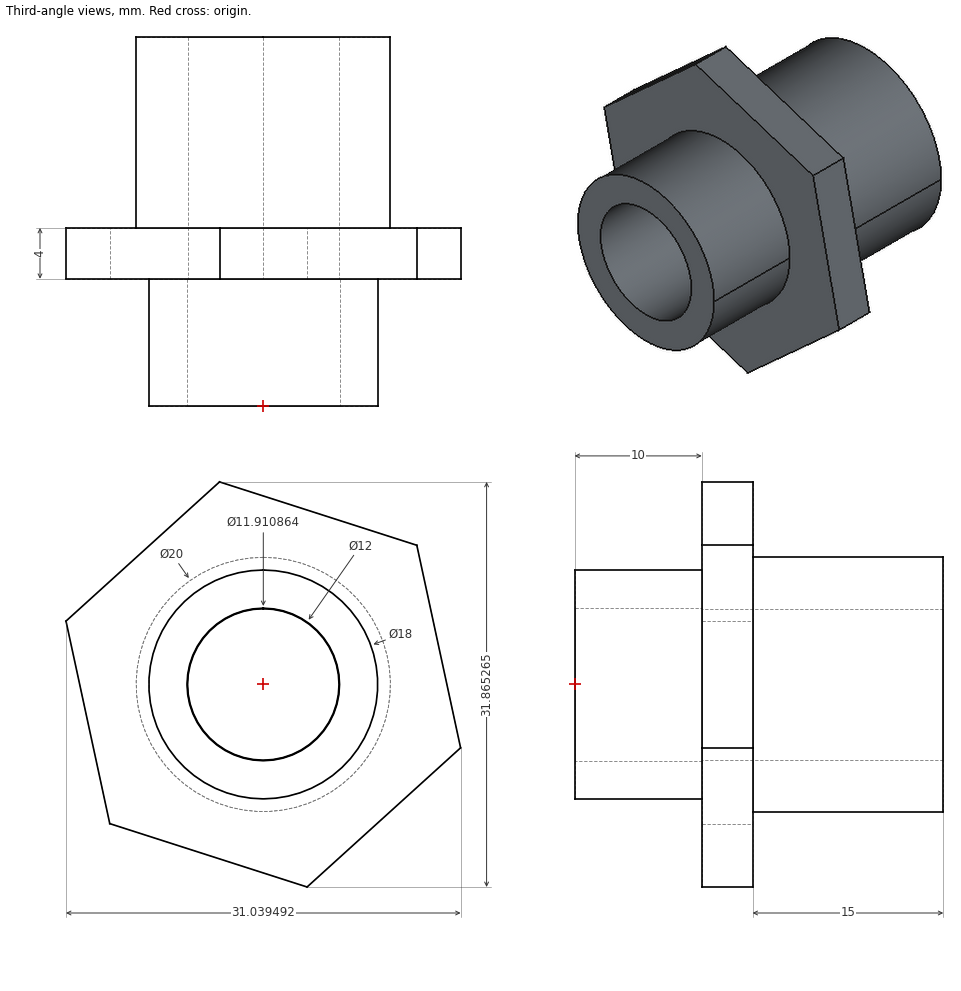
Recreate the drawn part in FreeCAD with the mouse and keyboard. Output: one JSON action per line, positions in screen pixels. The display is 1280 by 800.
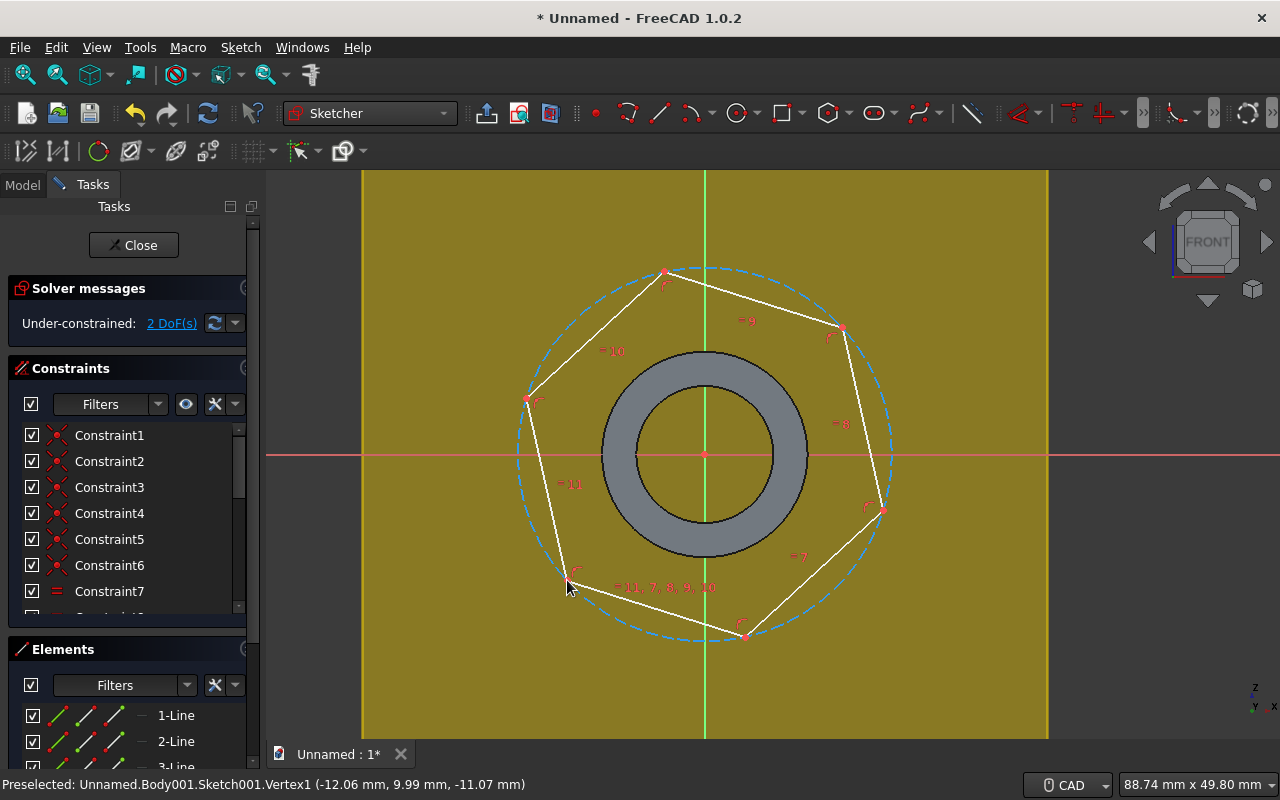
{"action": "left_click", "coordinate": [738, 114]}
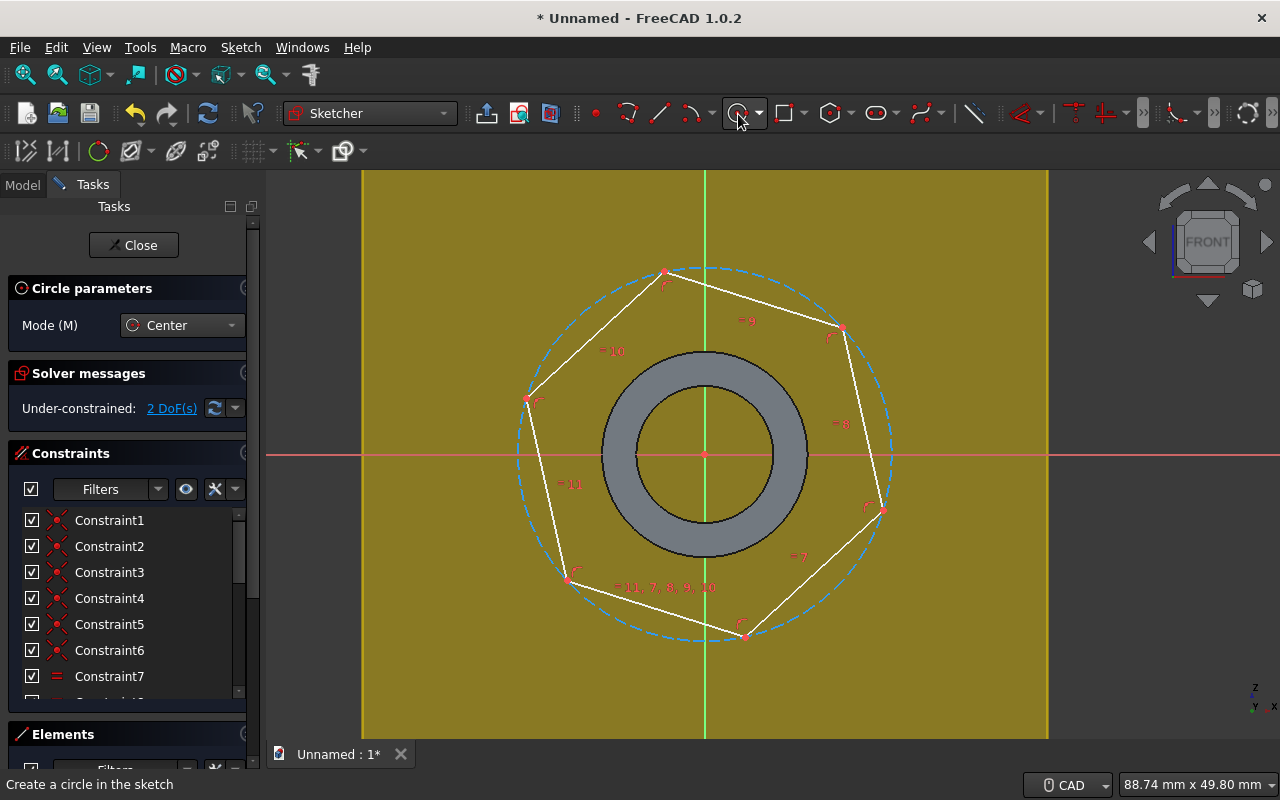
{"action": "left_click", "coordinate": [705, 455]}
{"action": "mouse_move", "coordinate": [753, 406]}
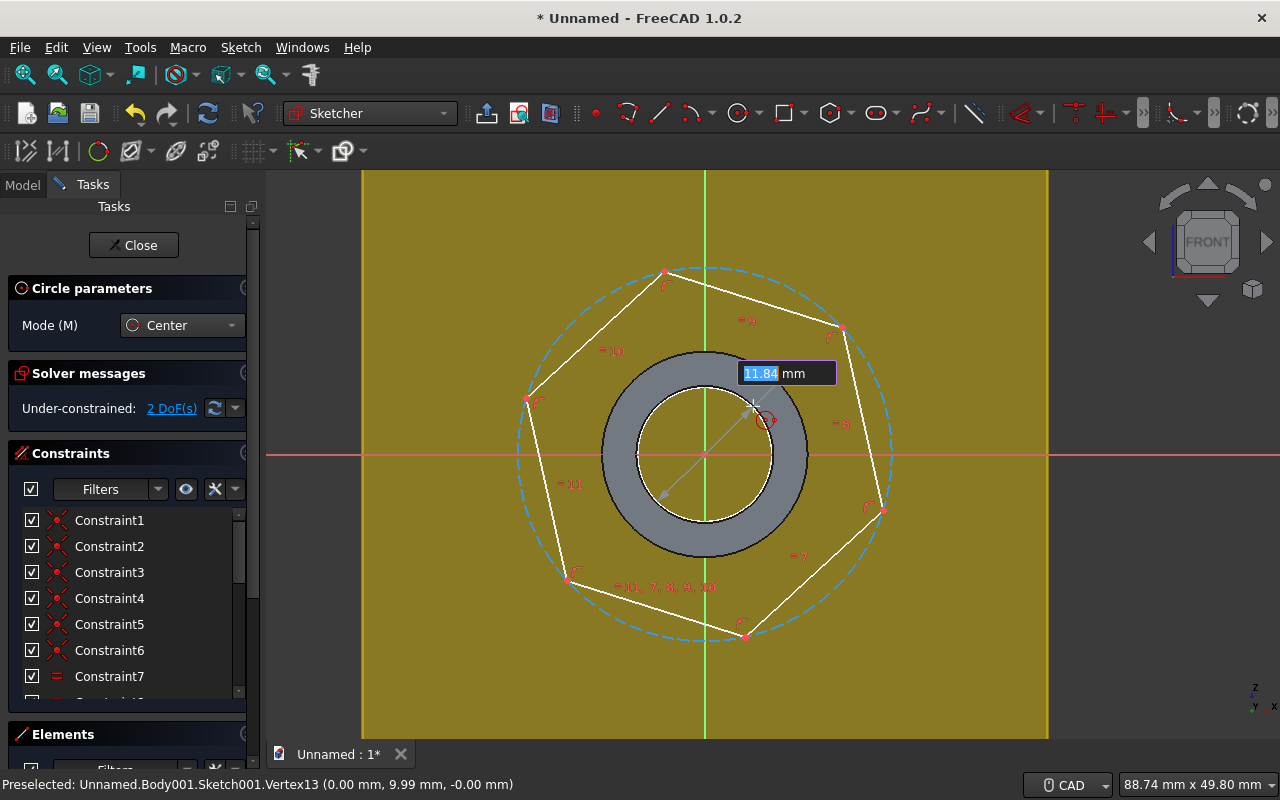
{"action": "type", "text": "11.910864"}
{"action": "key", "text": "Return"}
{"action": "key", "text": "Escape"}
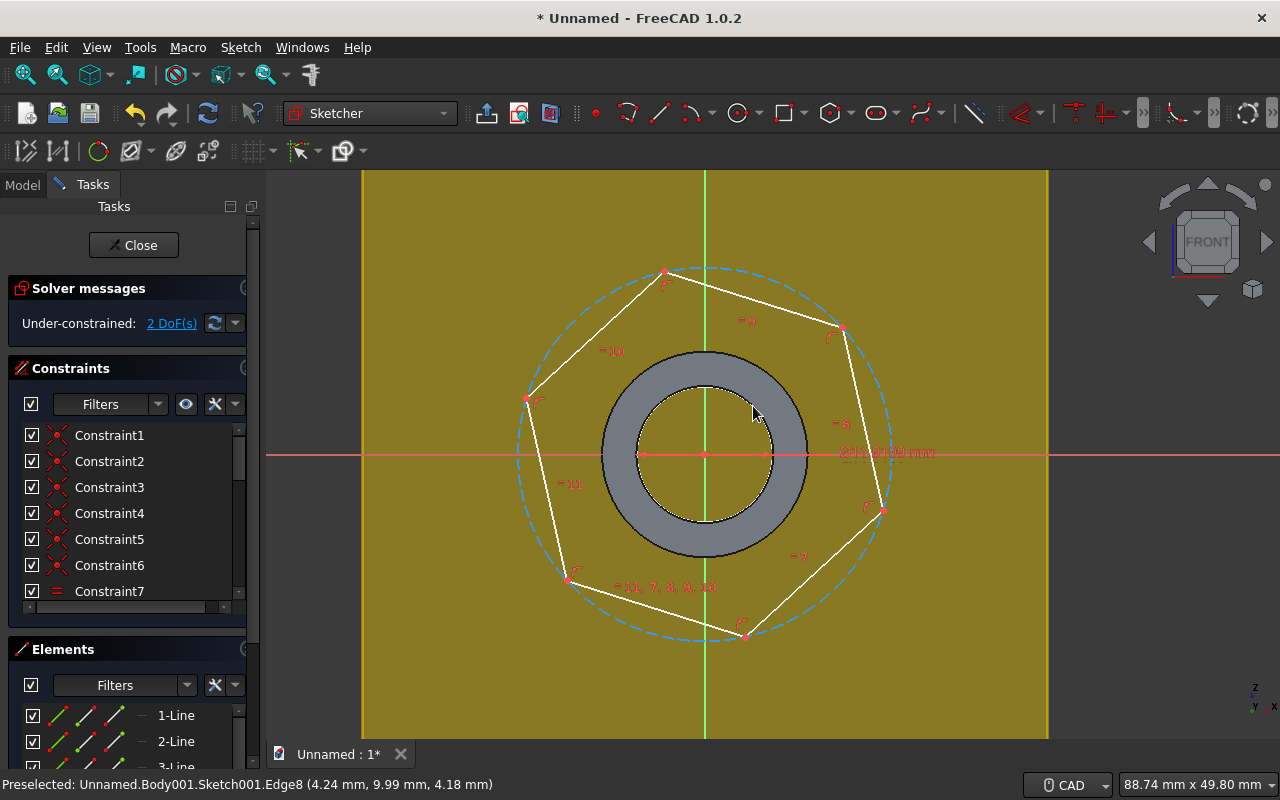
{"action": "left_click", "coordinate": [1020, 114]}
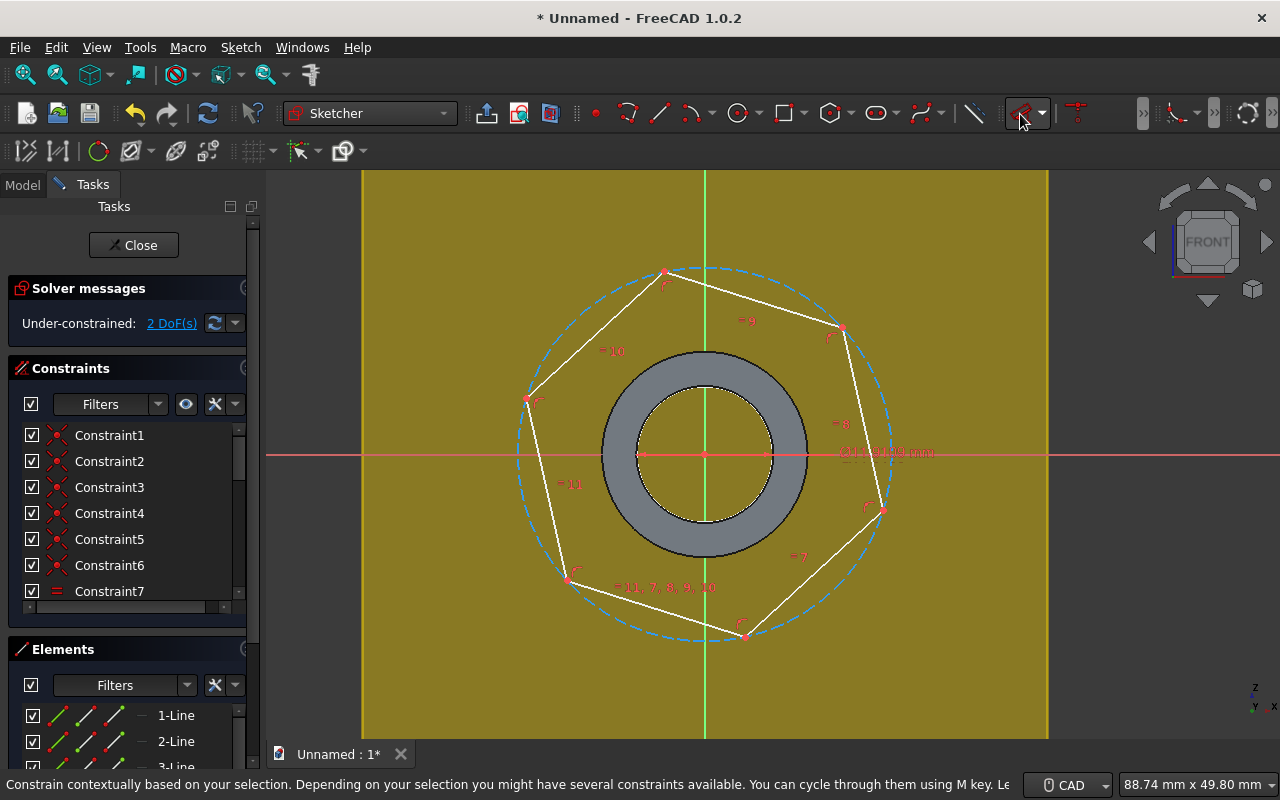
{"action": "left_click", "coordinate": [526, 398]}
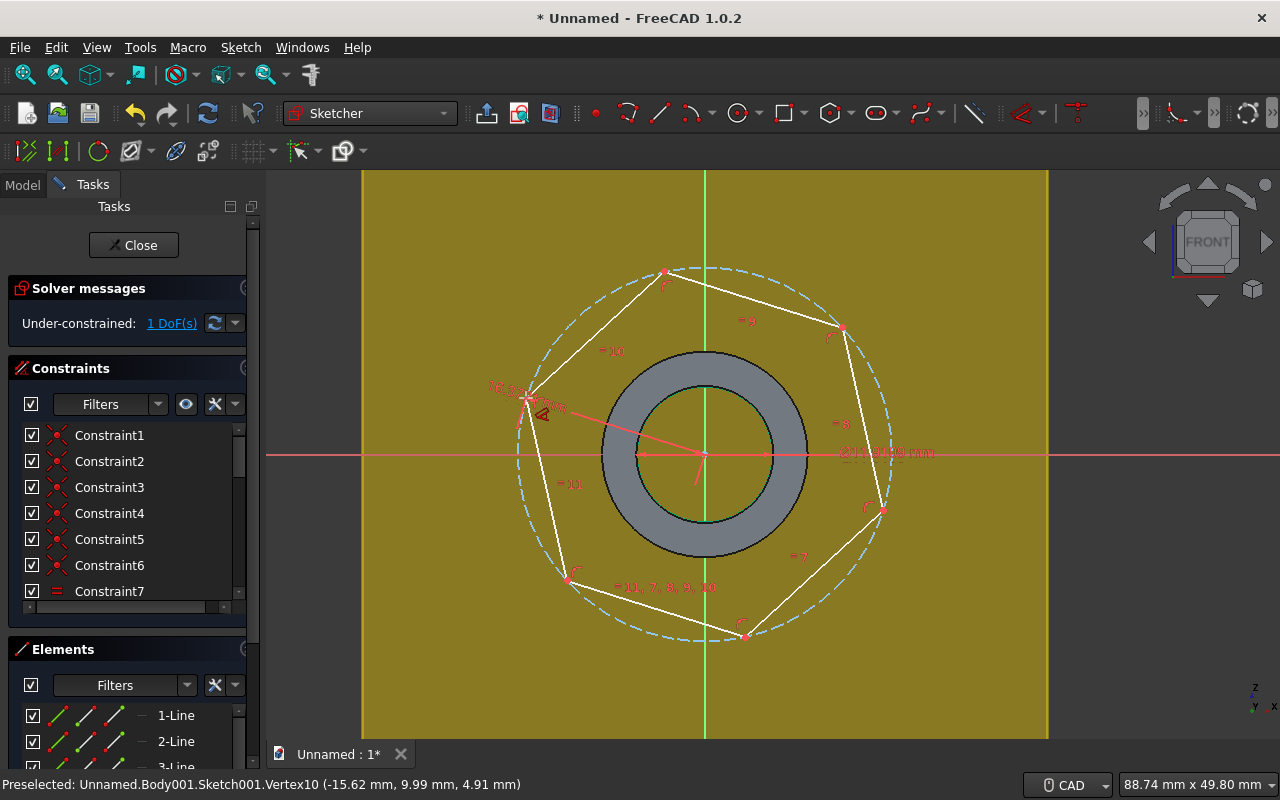
{"action": "left_click", "coordinate": [883, 511]}
{"action": "left_click", "coordinate": [623, 364]}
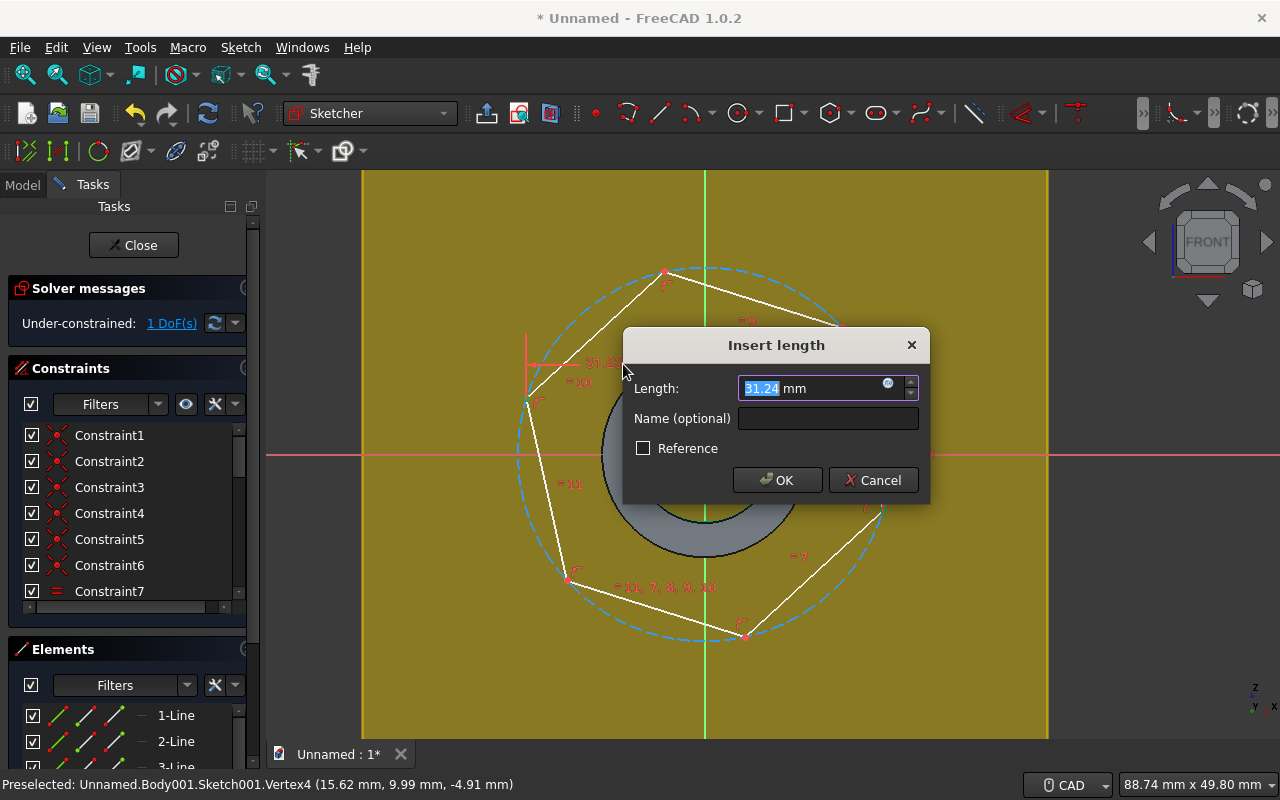
{"action": "type", "text": "31.039492"}
{"action": "key", "text": "Return"}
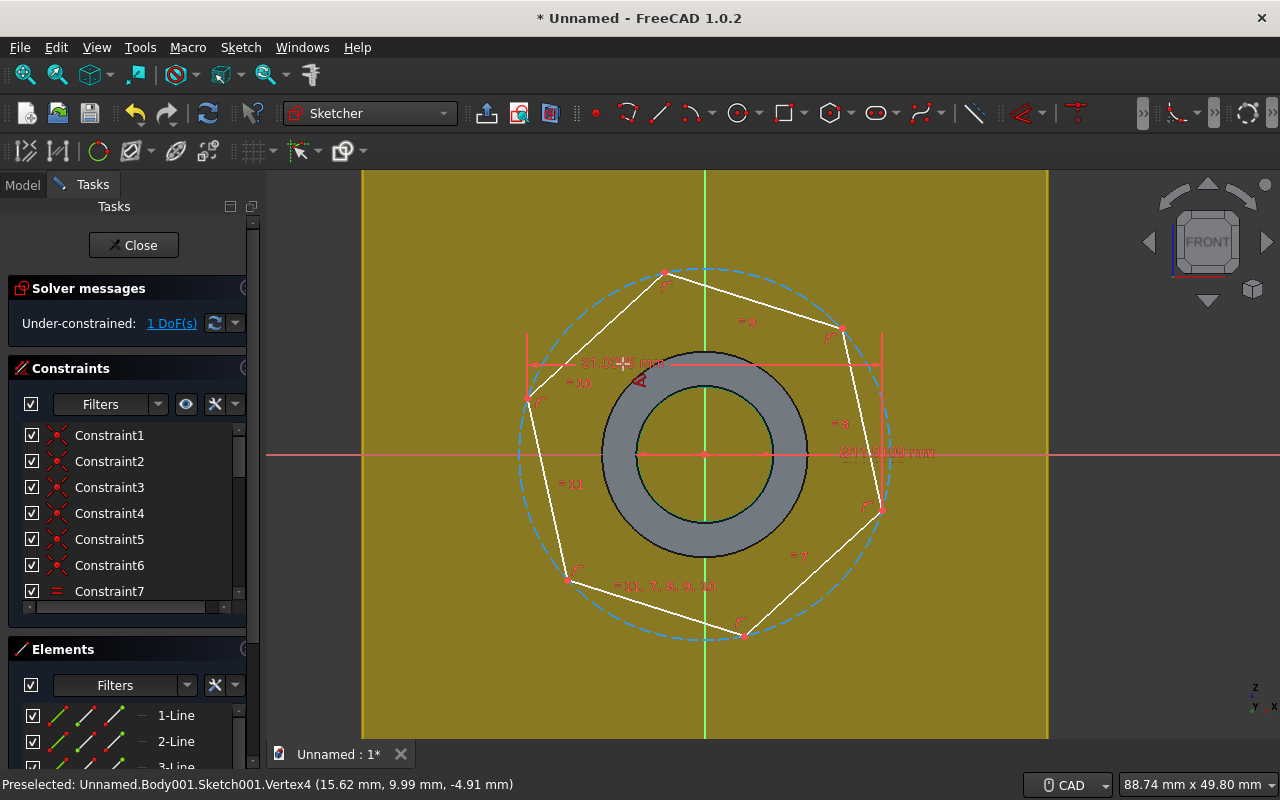
{"action": "left_click", "coordinate": [745, 636]}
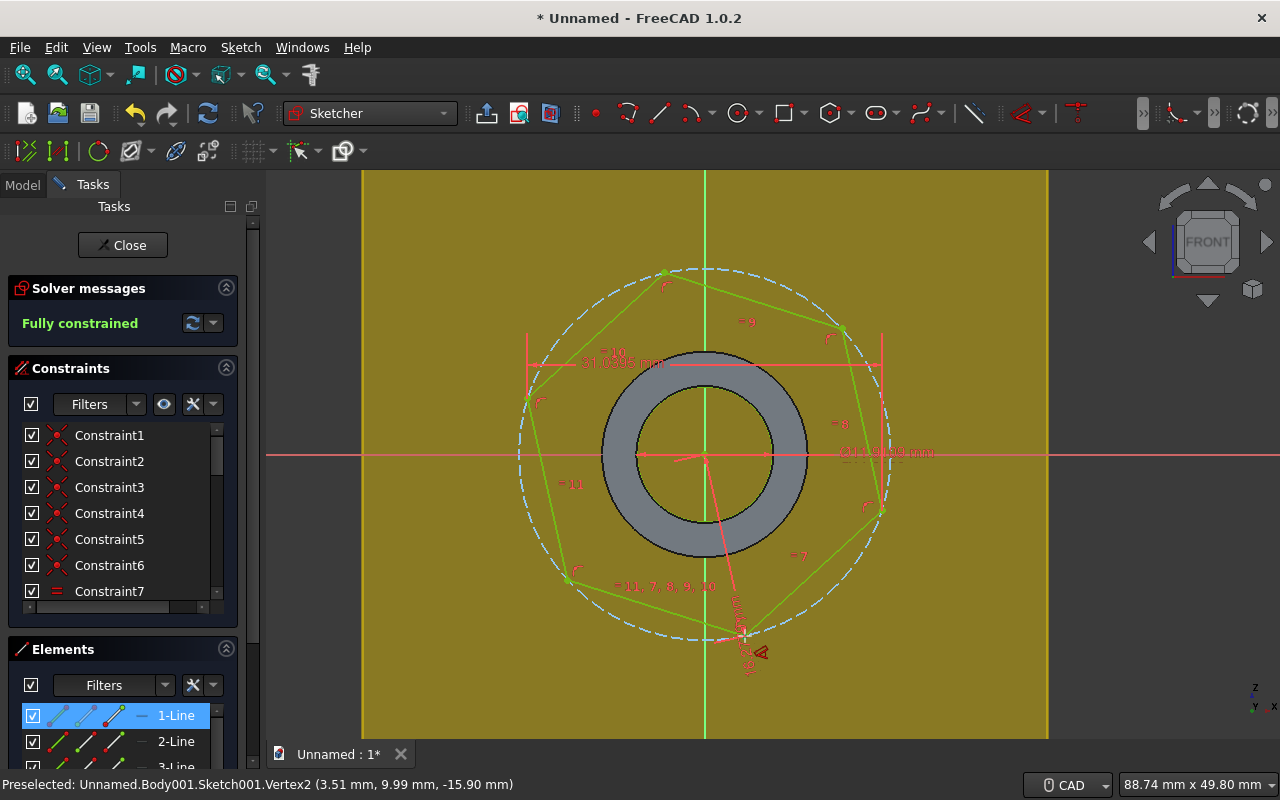
{"action": "left_click", "coordinate": [665, 273]}
{"action": "left_click", "coordinate": [779, 371]}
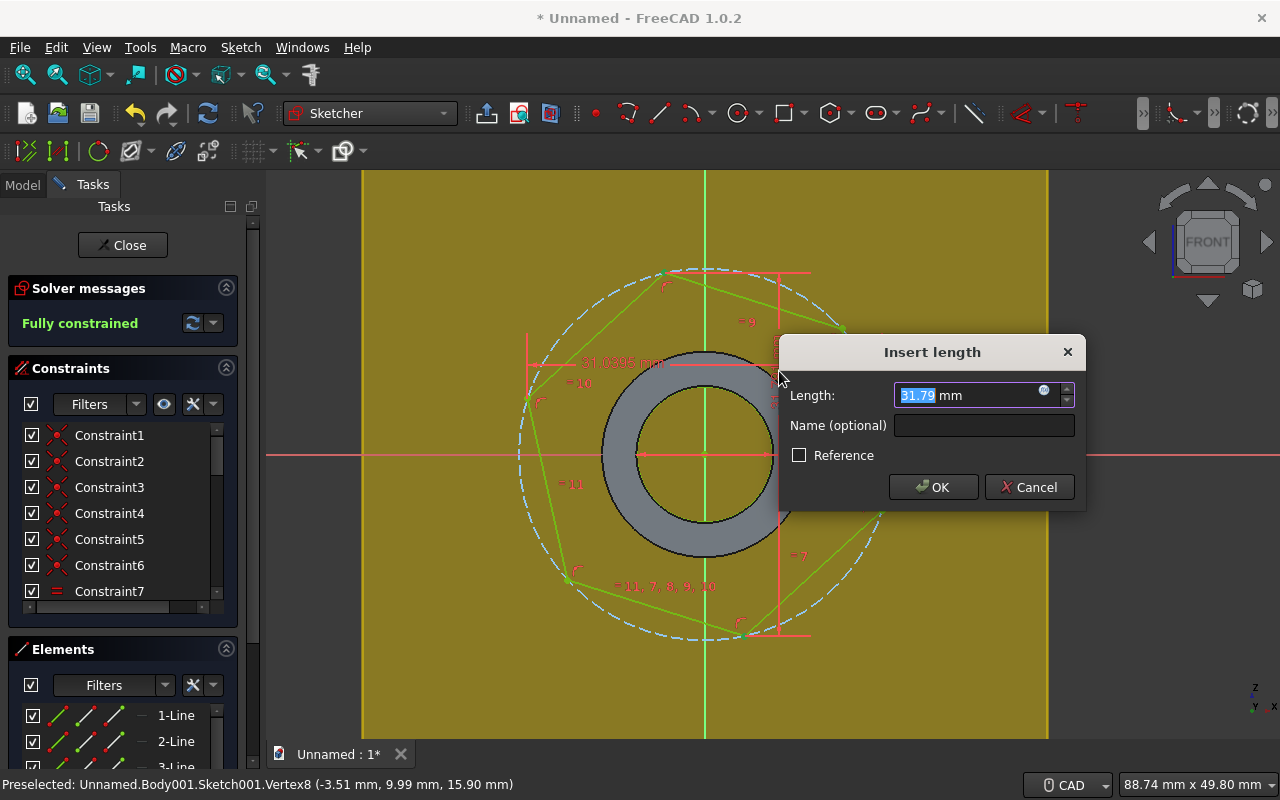
{"action": "type", "text": "31.865265"}
{"action": "key", "text": "Return"}
{"action": "key", "text": "Escape"}